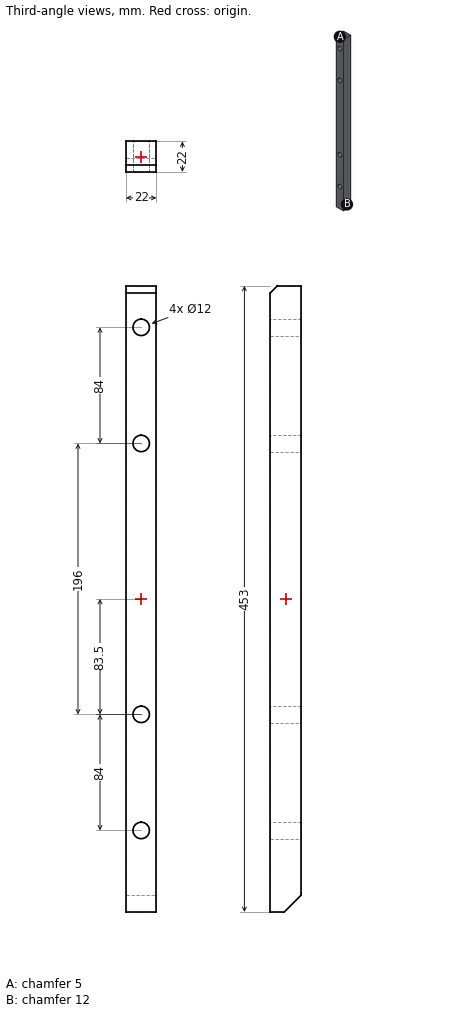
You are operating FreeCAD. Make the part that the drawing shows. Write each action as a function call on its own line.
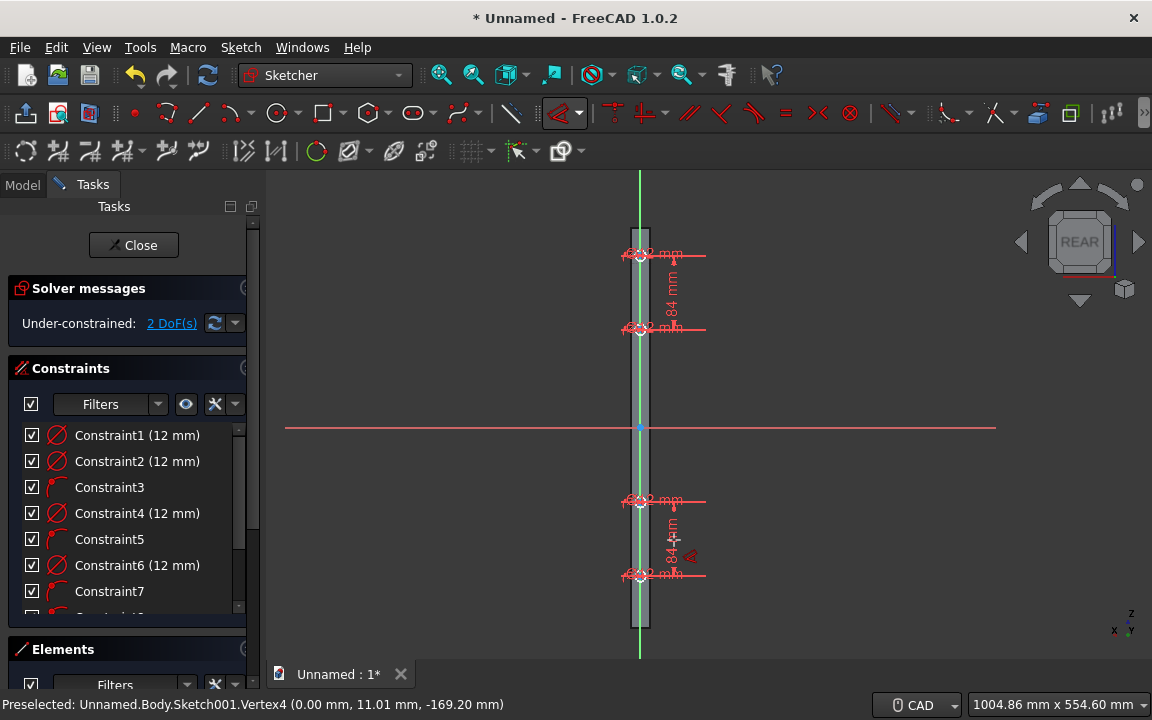
click(640, 502)
click(674, 465)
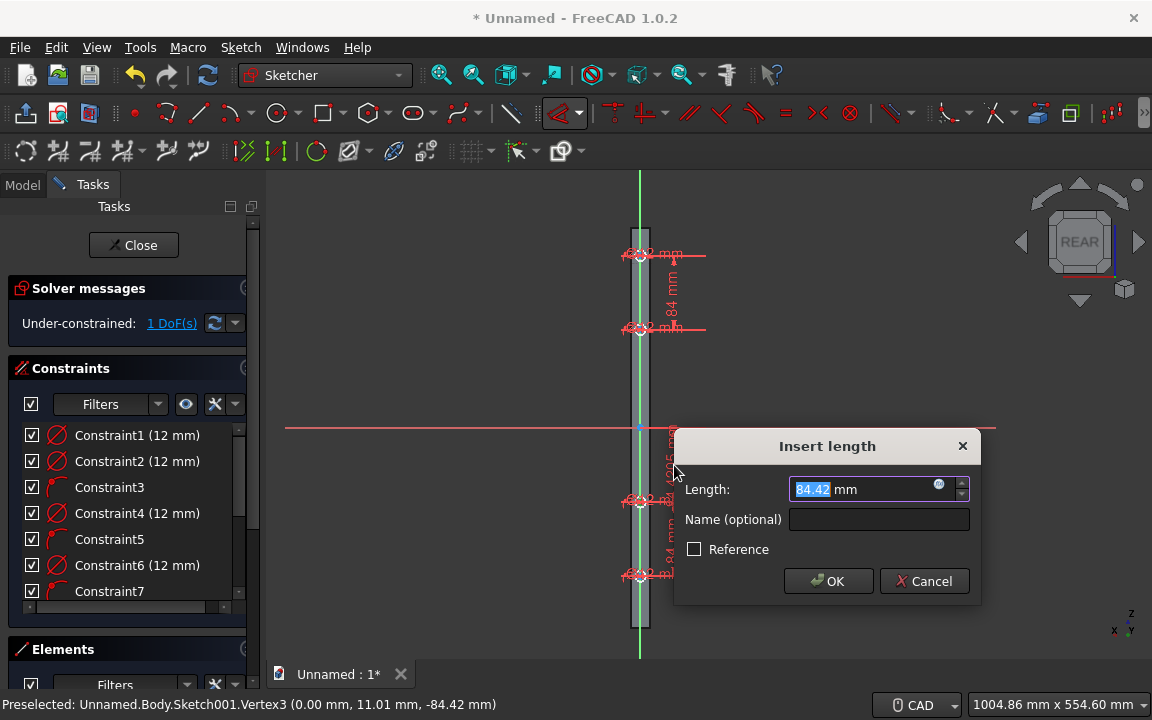
text(83.5)
key(Return)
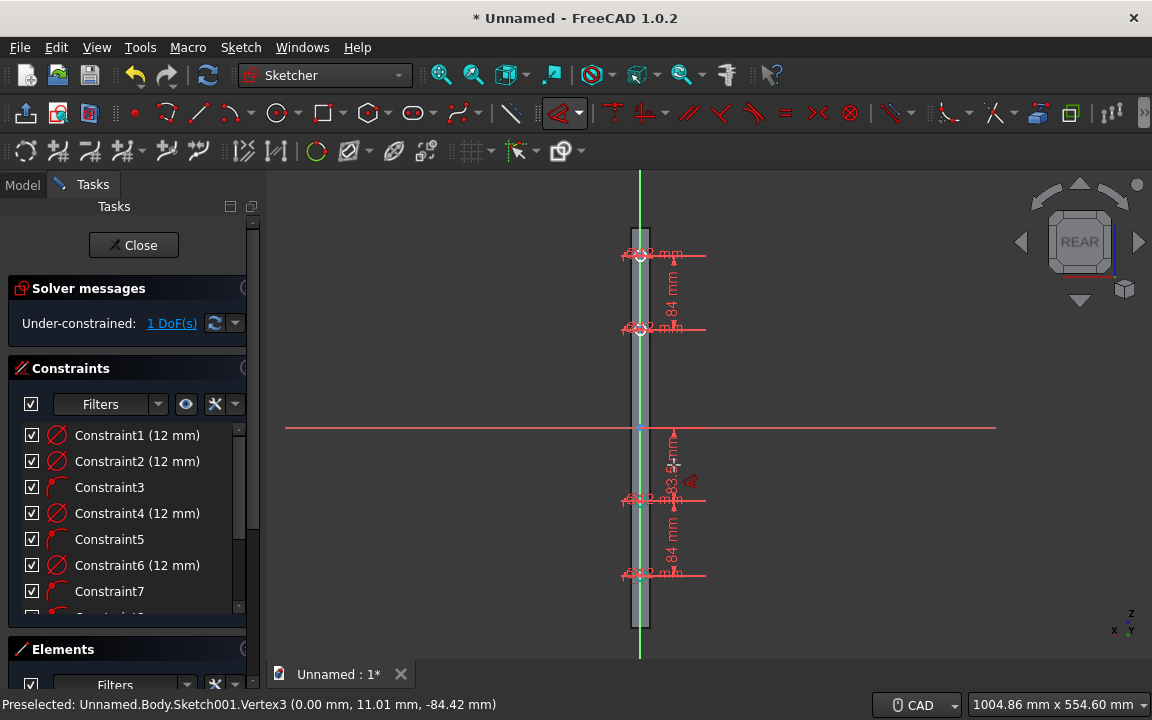
click(640, 330)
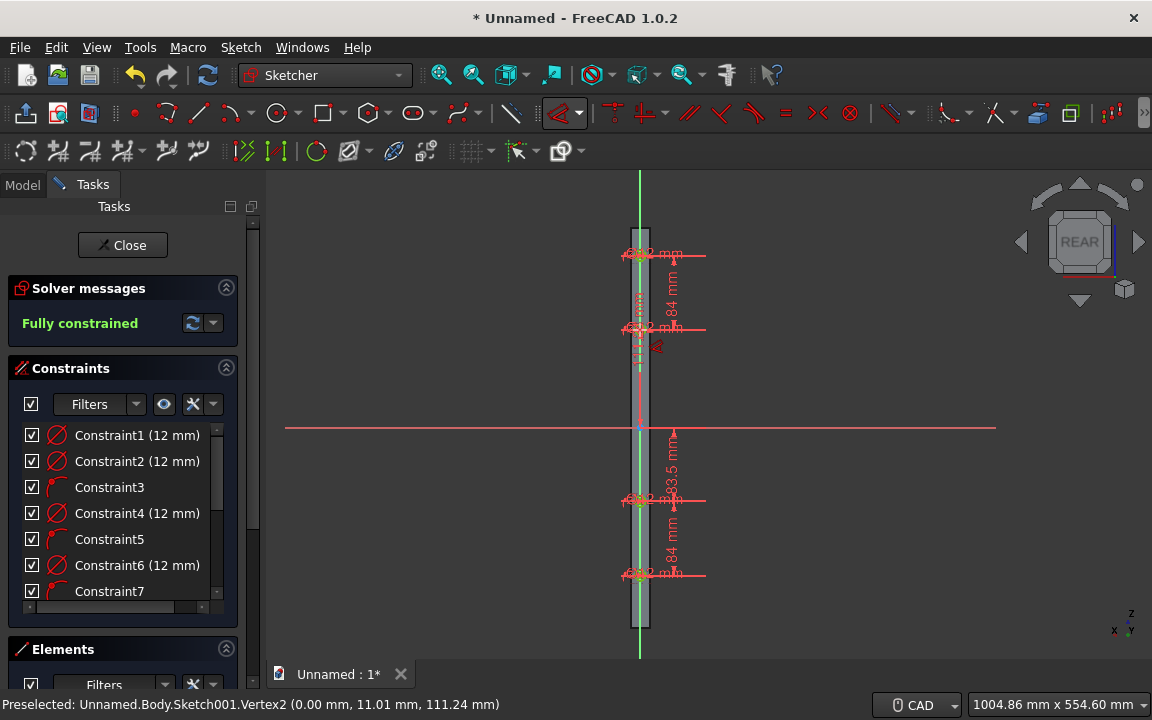
click(640, 501)
click(674, 376)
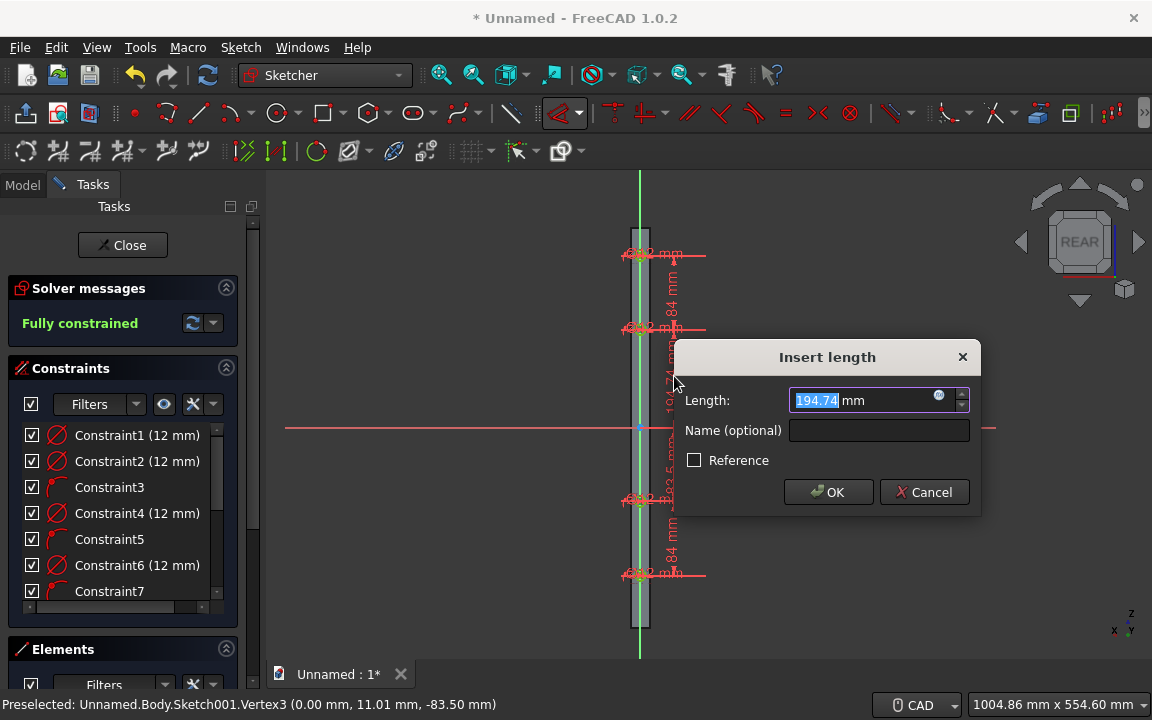
text(196)
key(Return)
key(Escape)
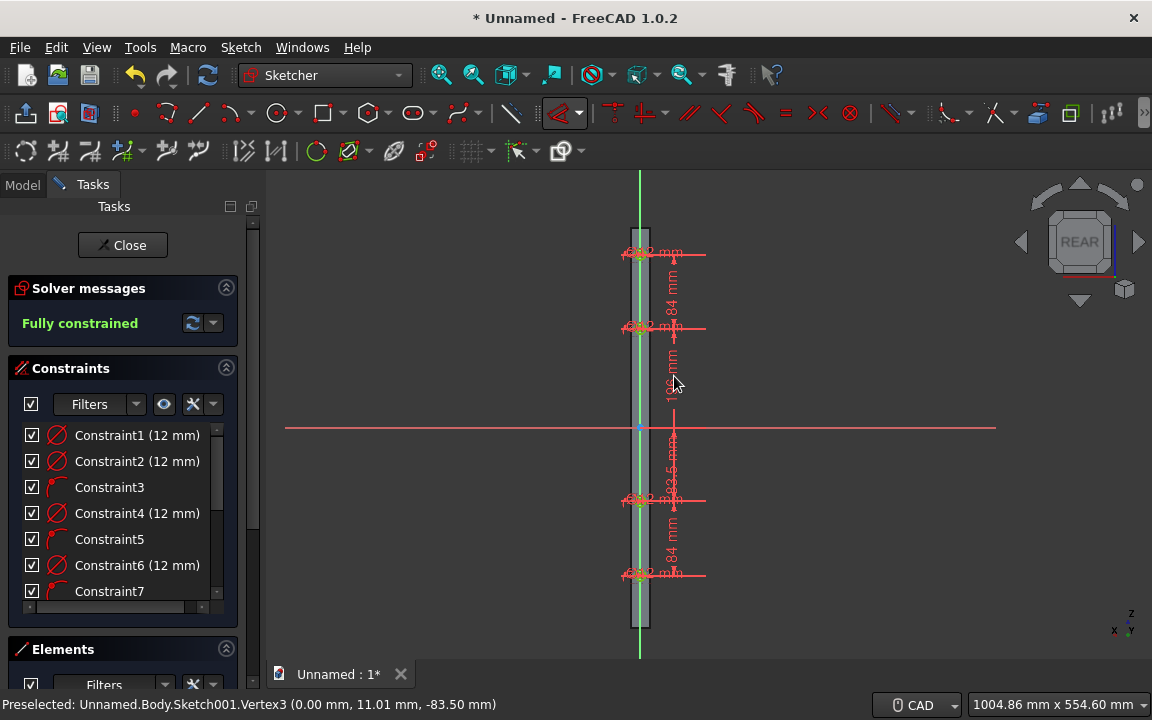
click(123, 245)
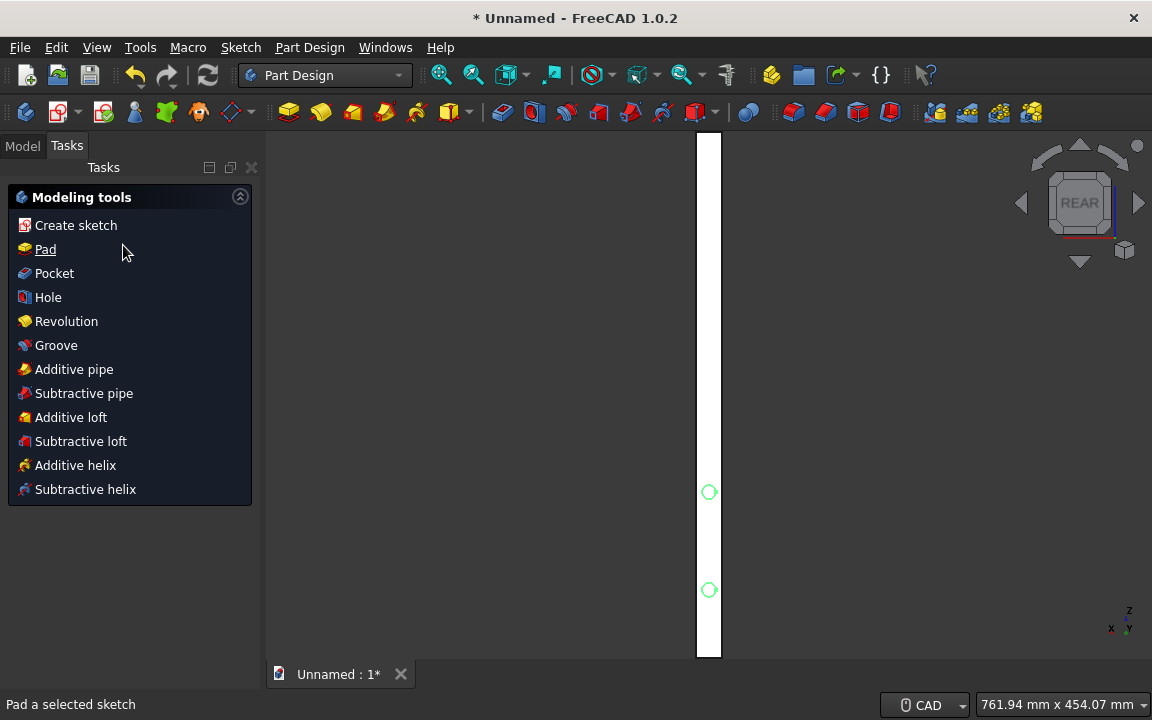
click(504, 112)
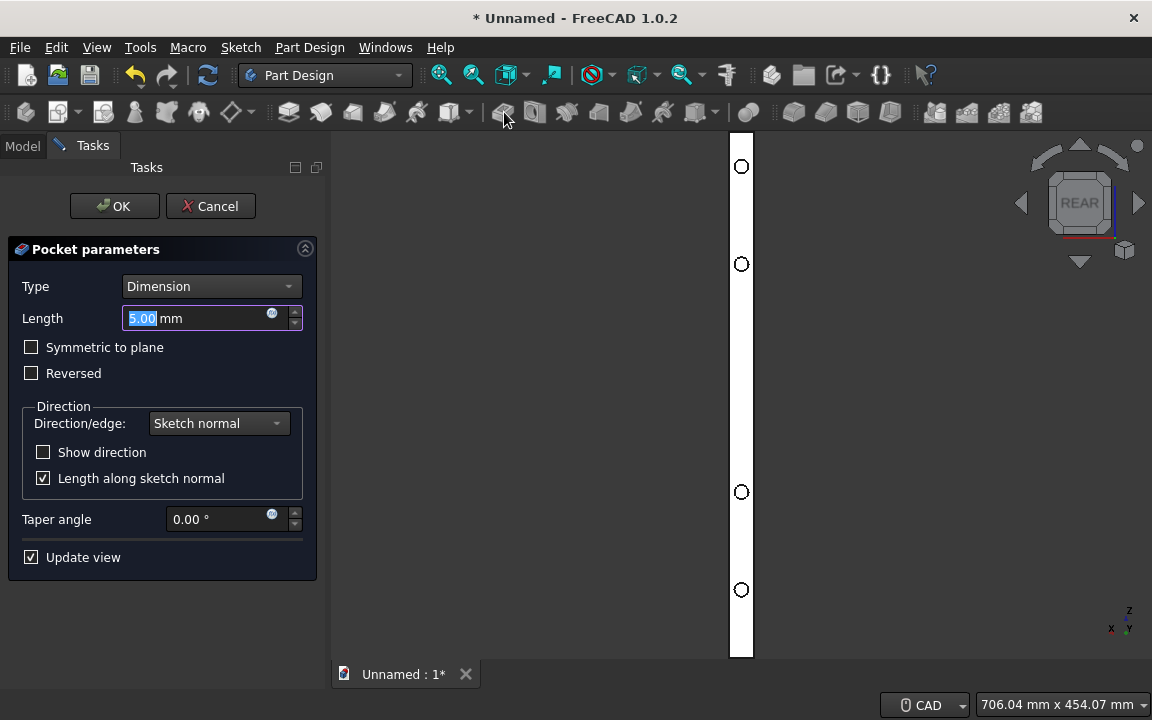
click(212, 286)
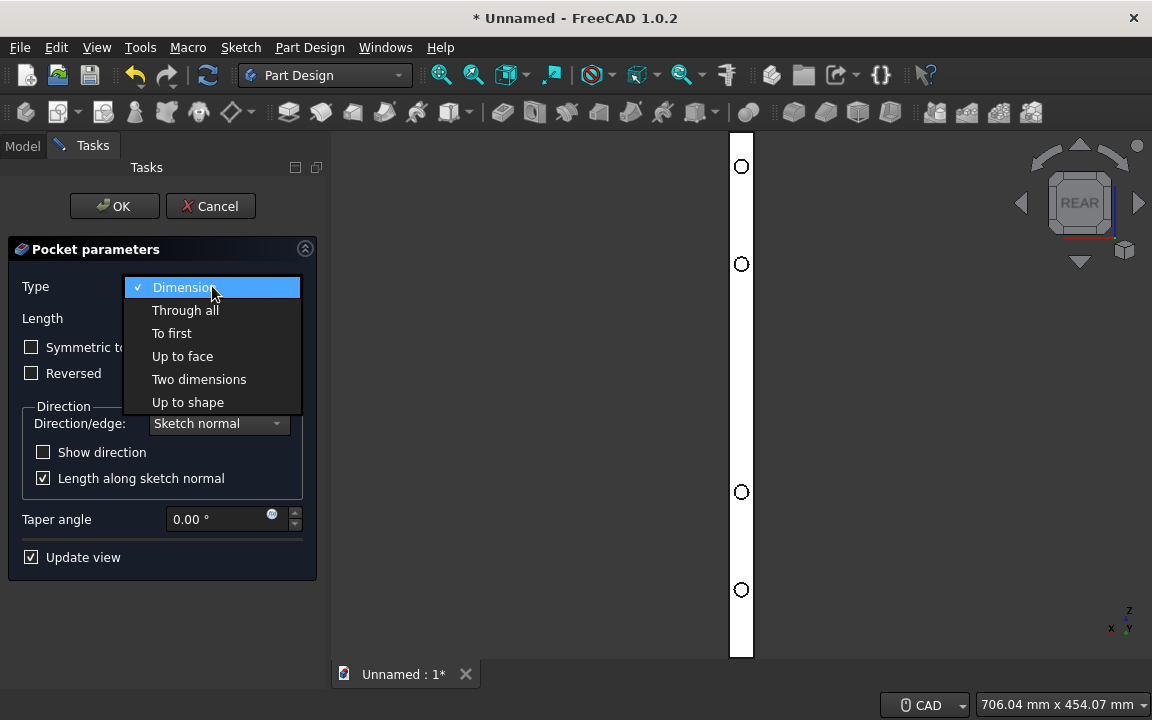
click(212, 310)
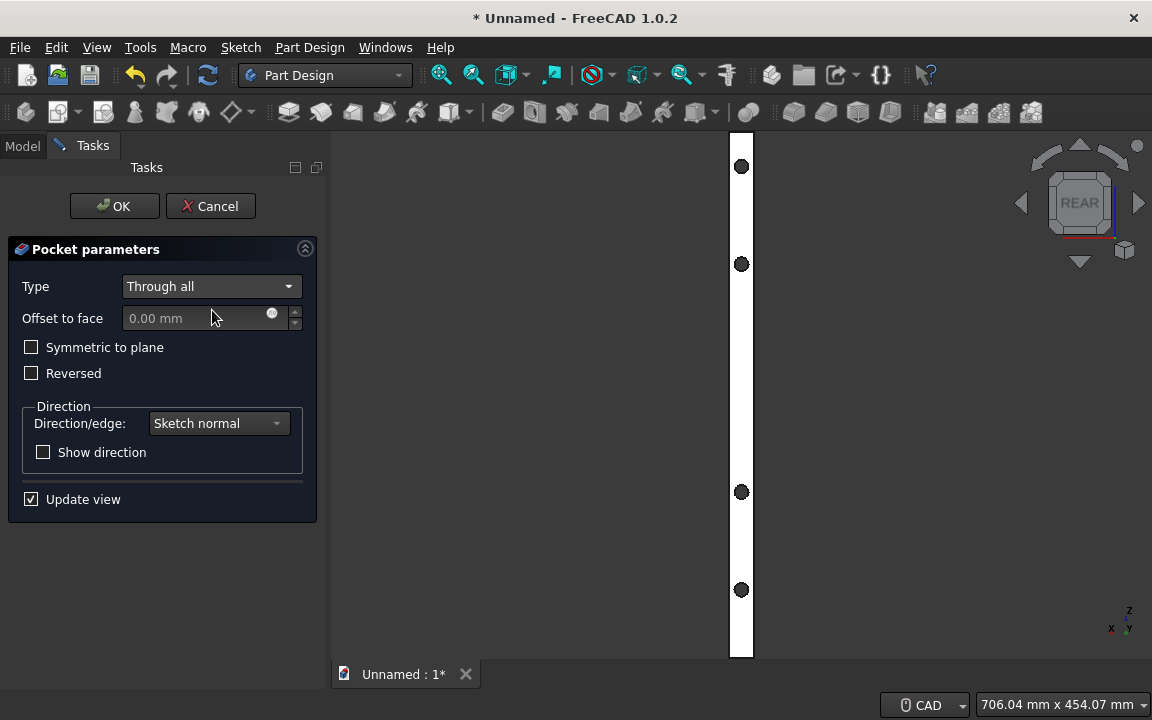
click(115, 206)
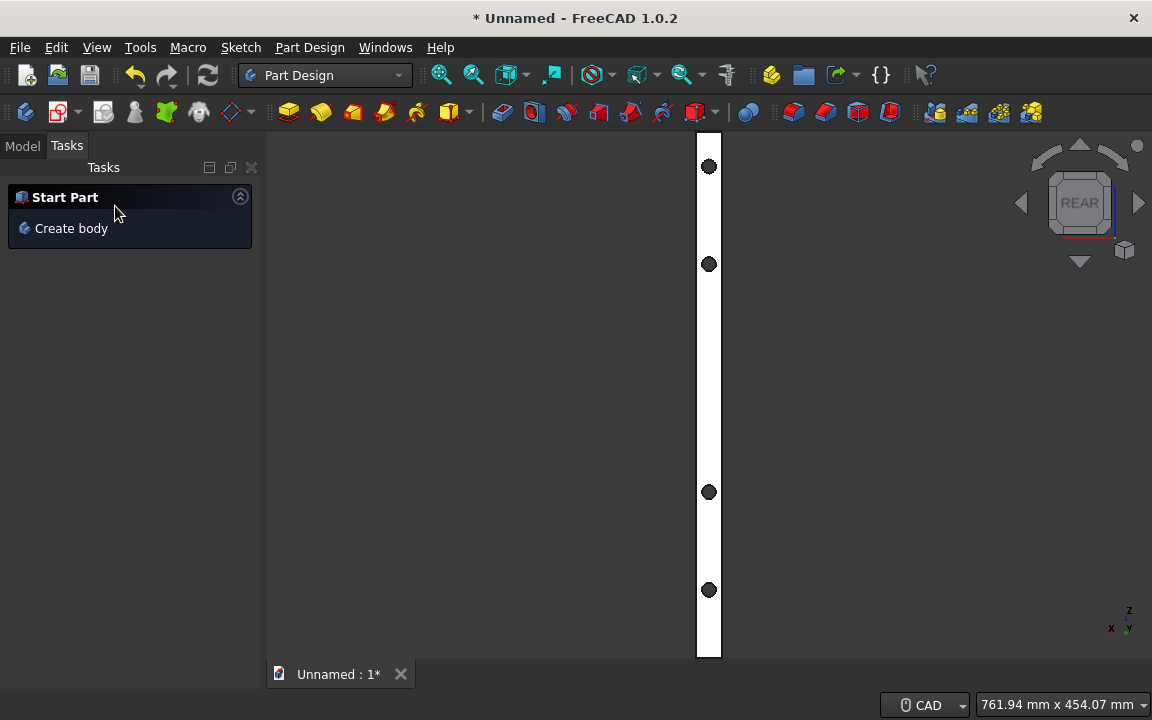
key(0)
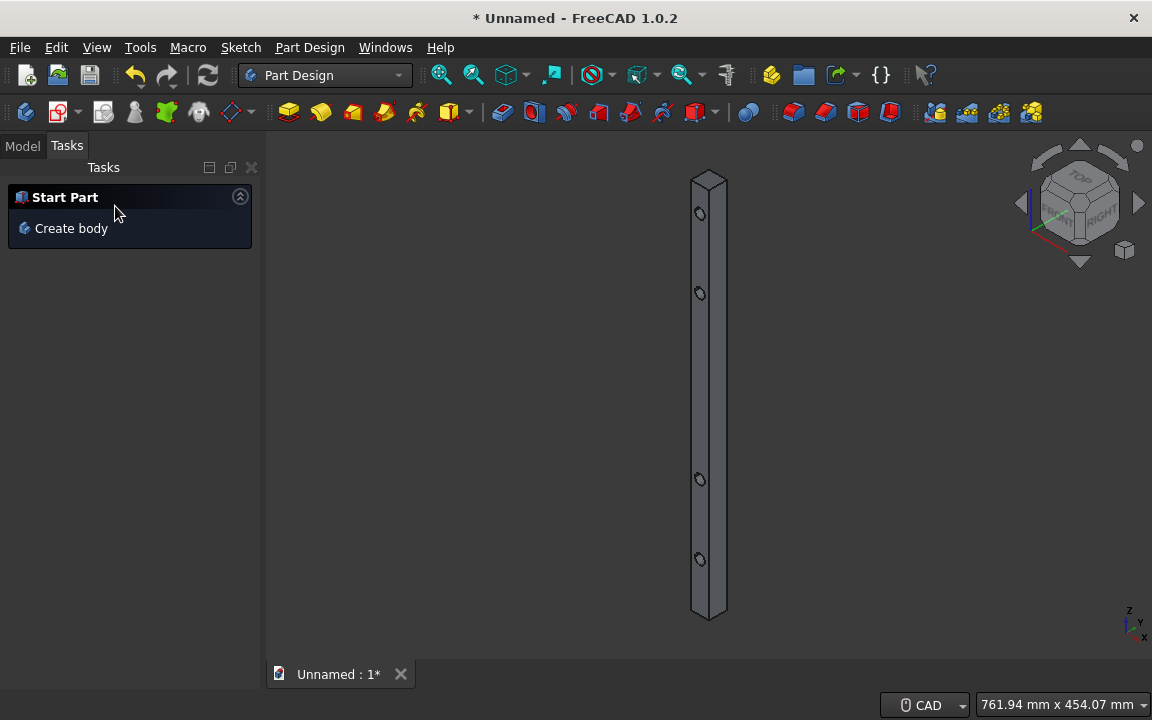
click(700, 184)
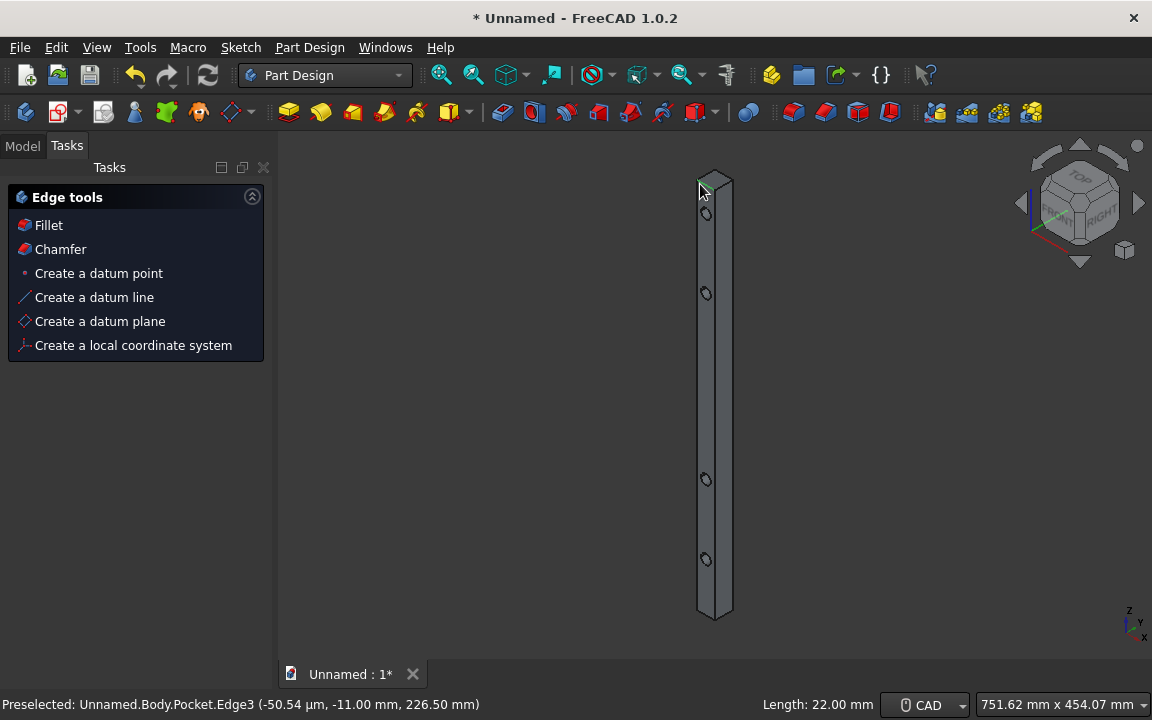
click(826, 112)